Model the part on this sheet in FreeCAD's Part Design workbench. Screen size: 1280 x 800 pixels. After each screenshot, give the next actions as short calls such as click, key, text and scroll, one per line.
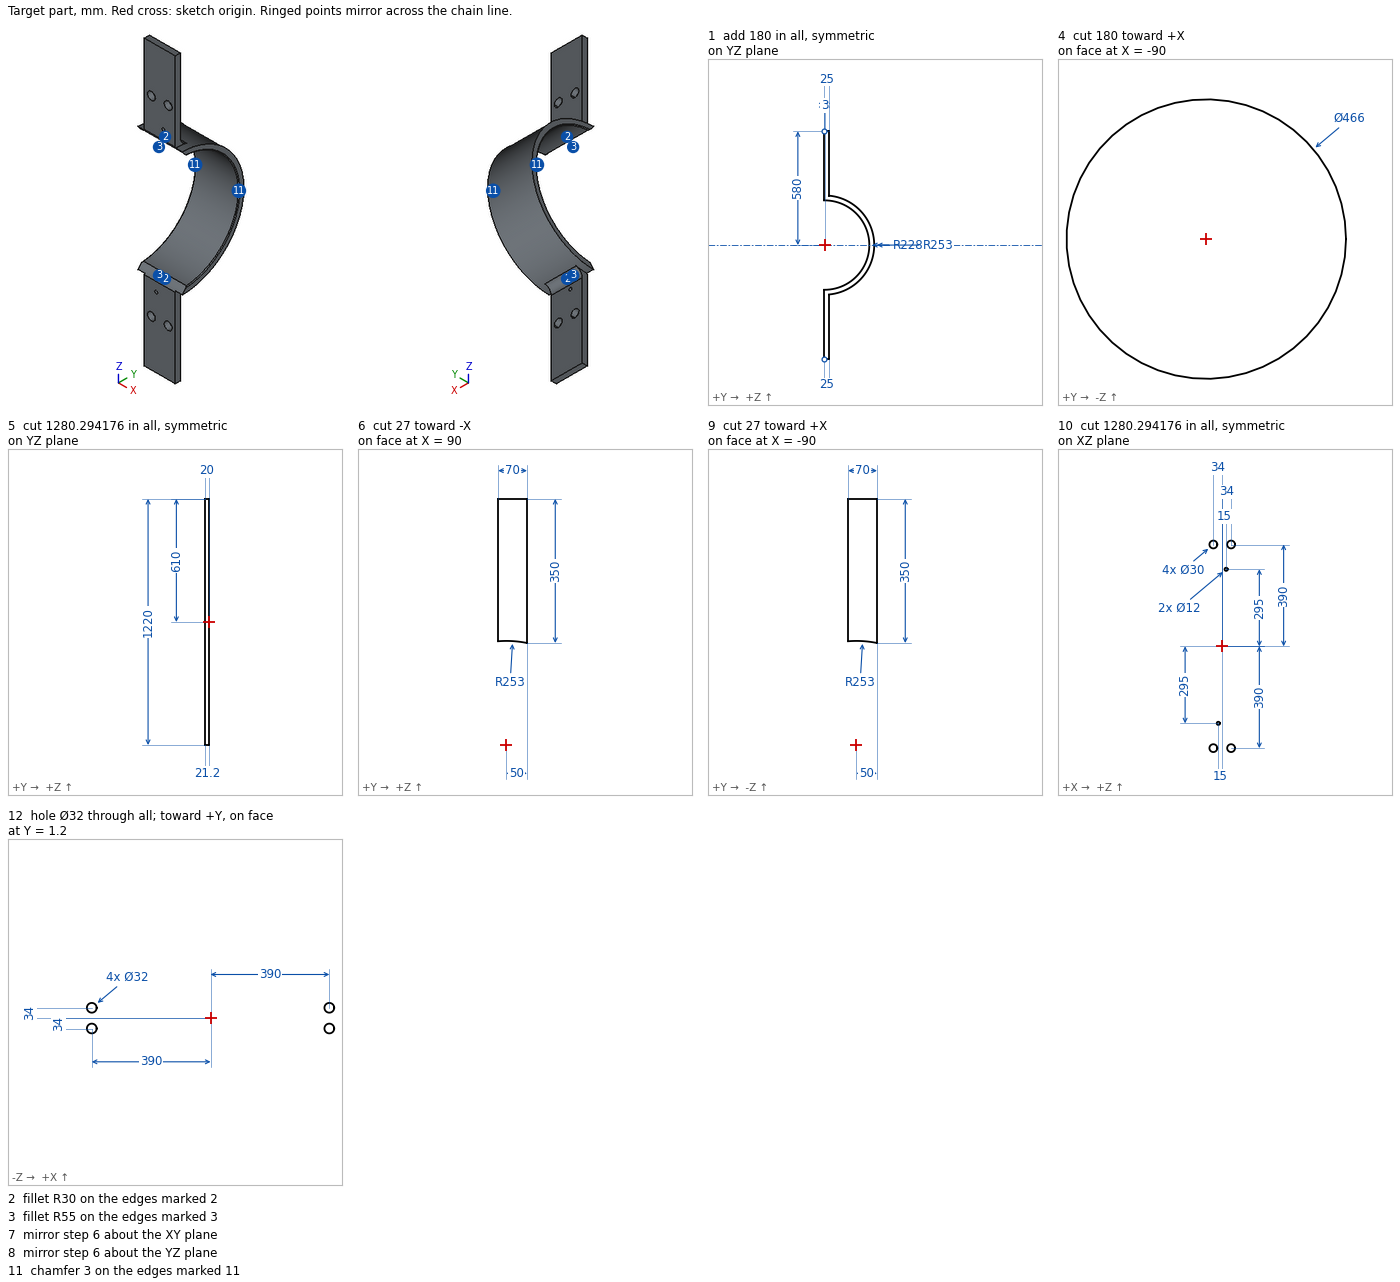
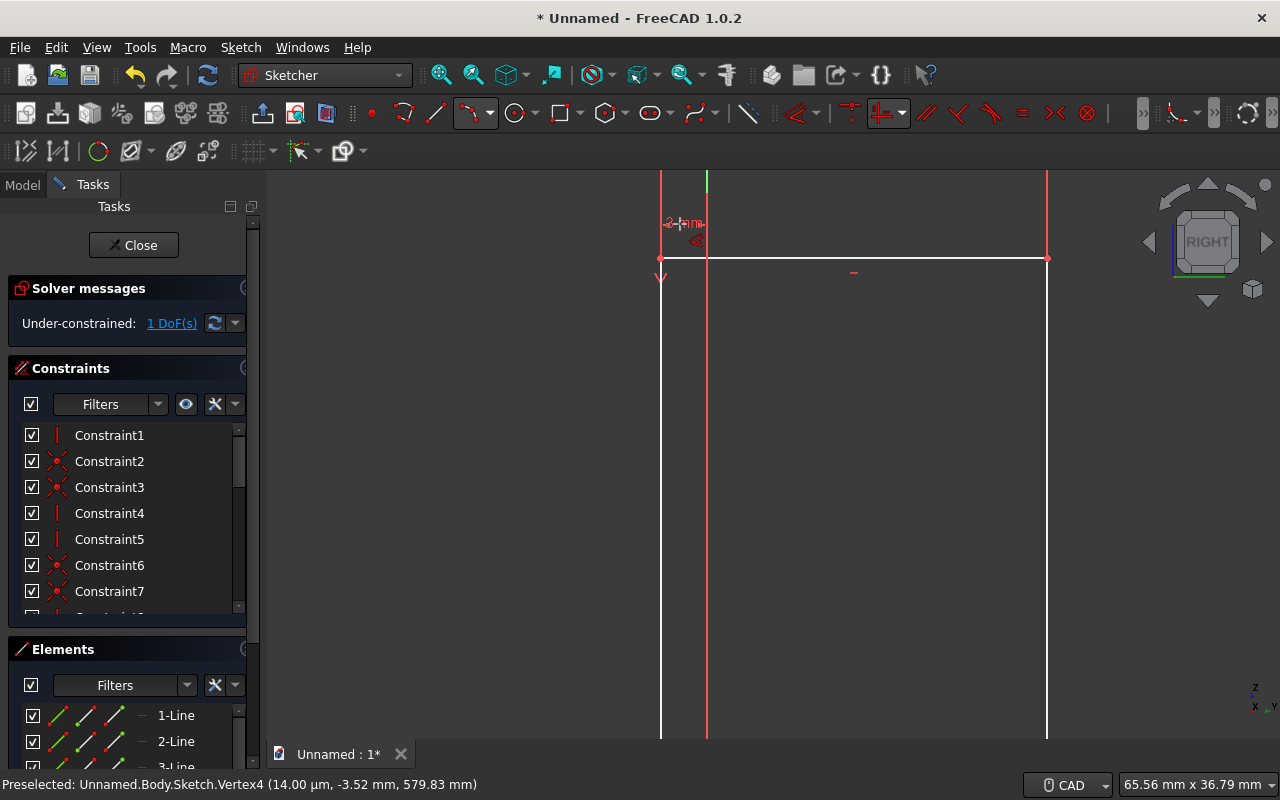
scroll(704, 454, down, 15)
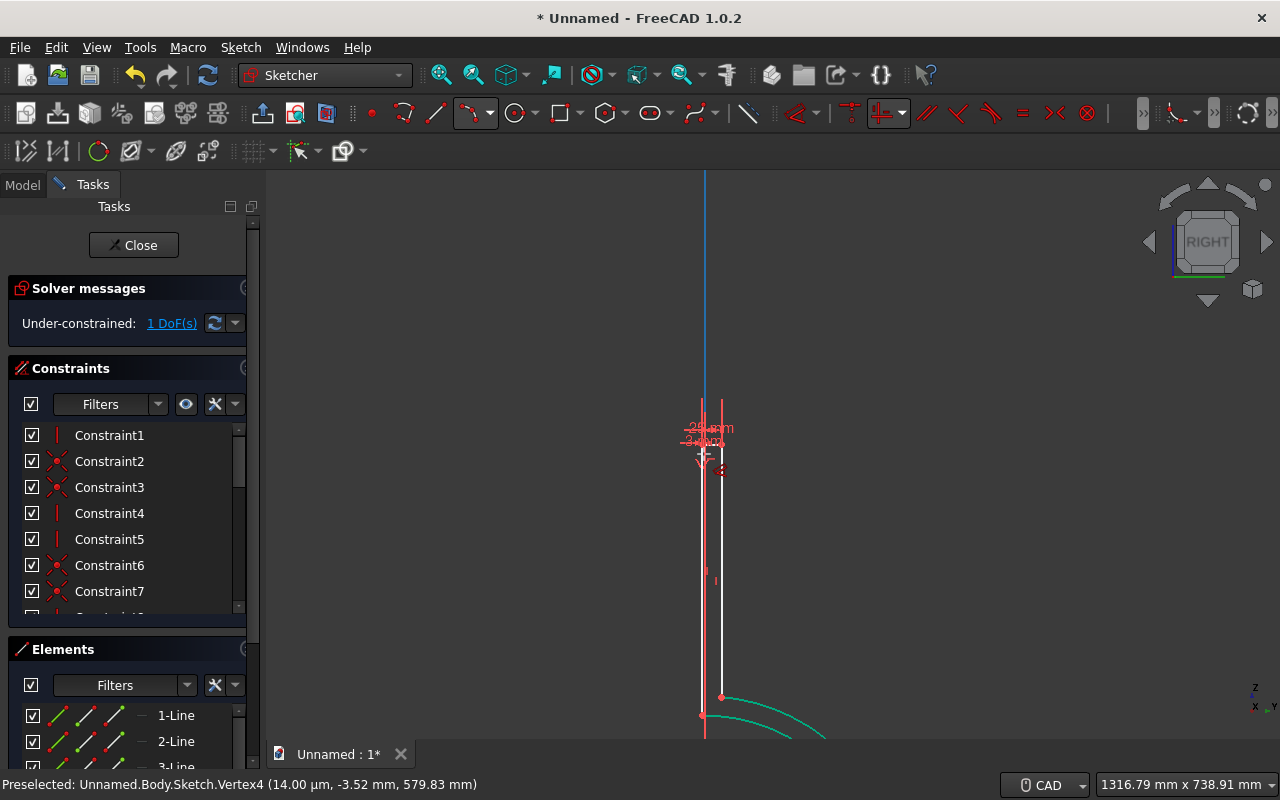
scroll(648, 200, down, 5)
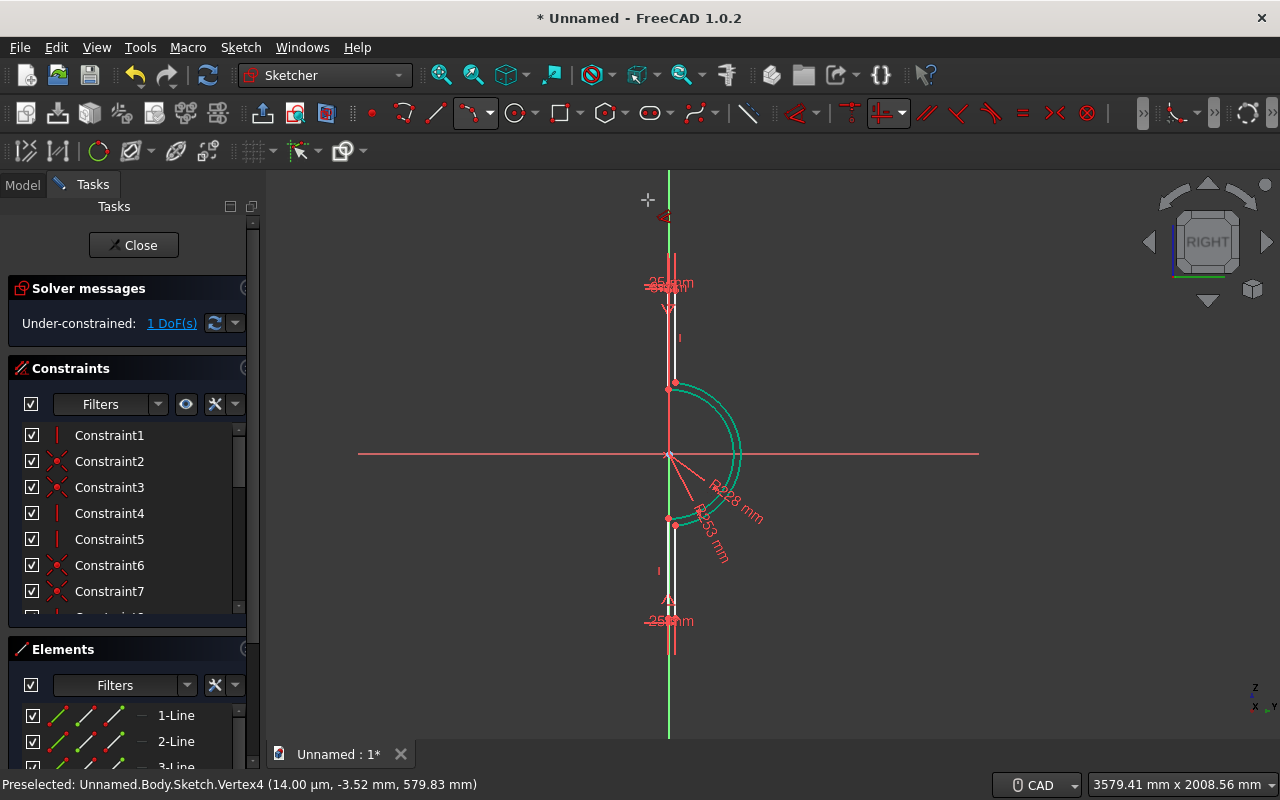
scroll(675, 290, up, 3)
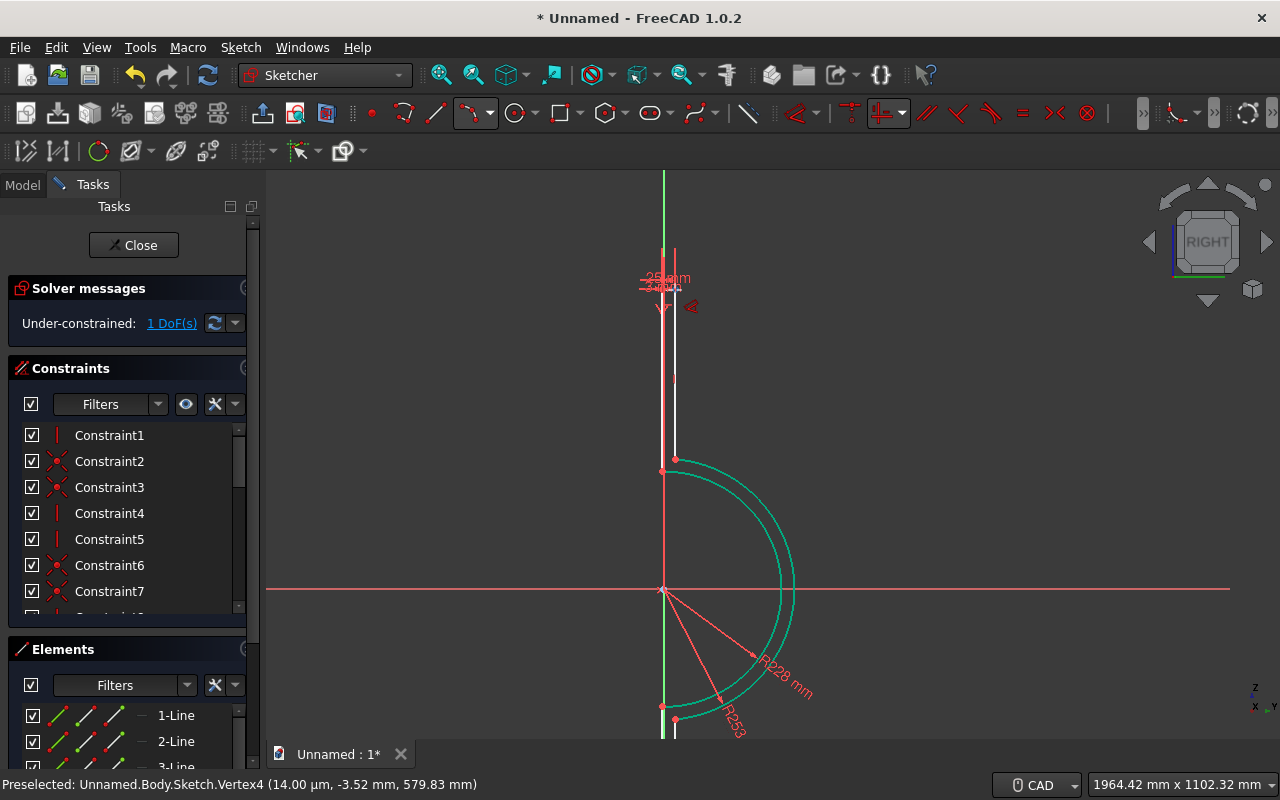
click(675, 290)
click(630, 440)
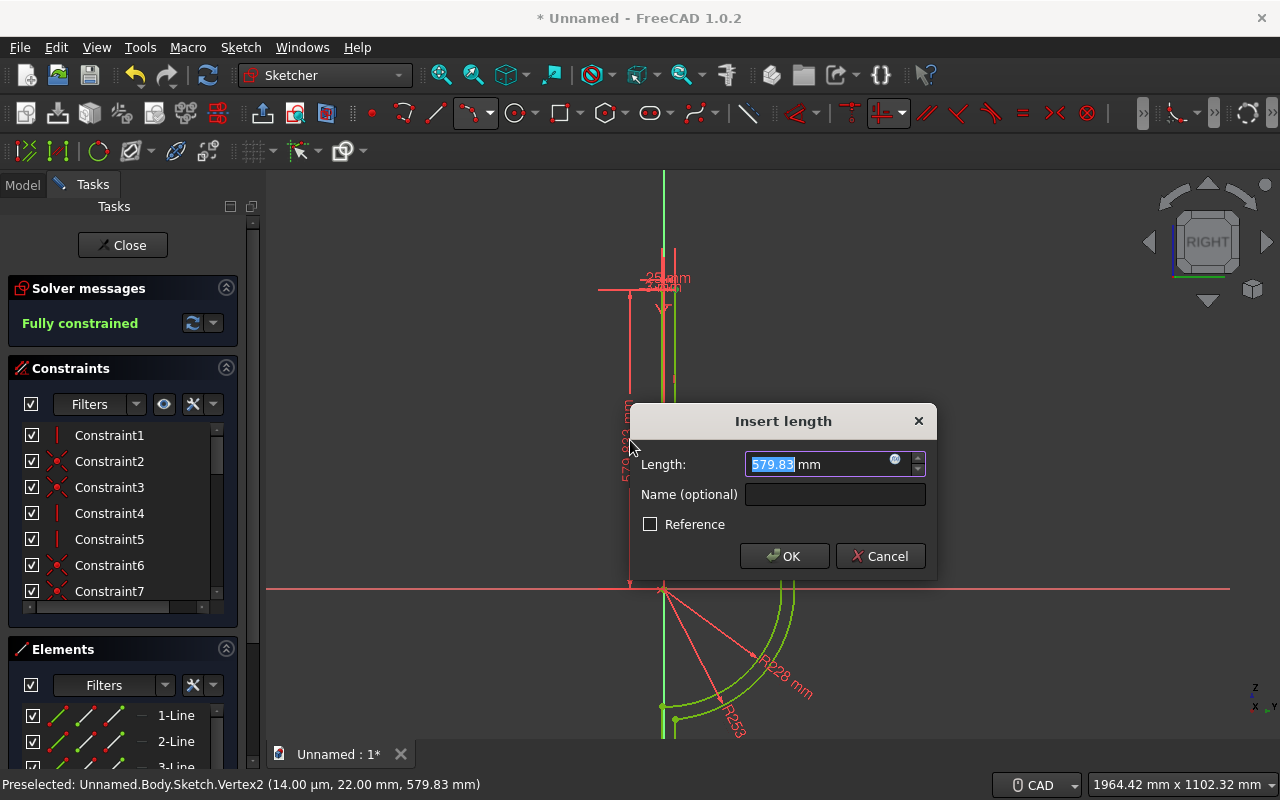
text(580)
key(Return)
key(Escape)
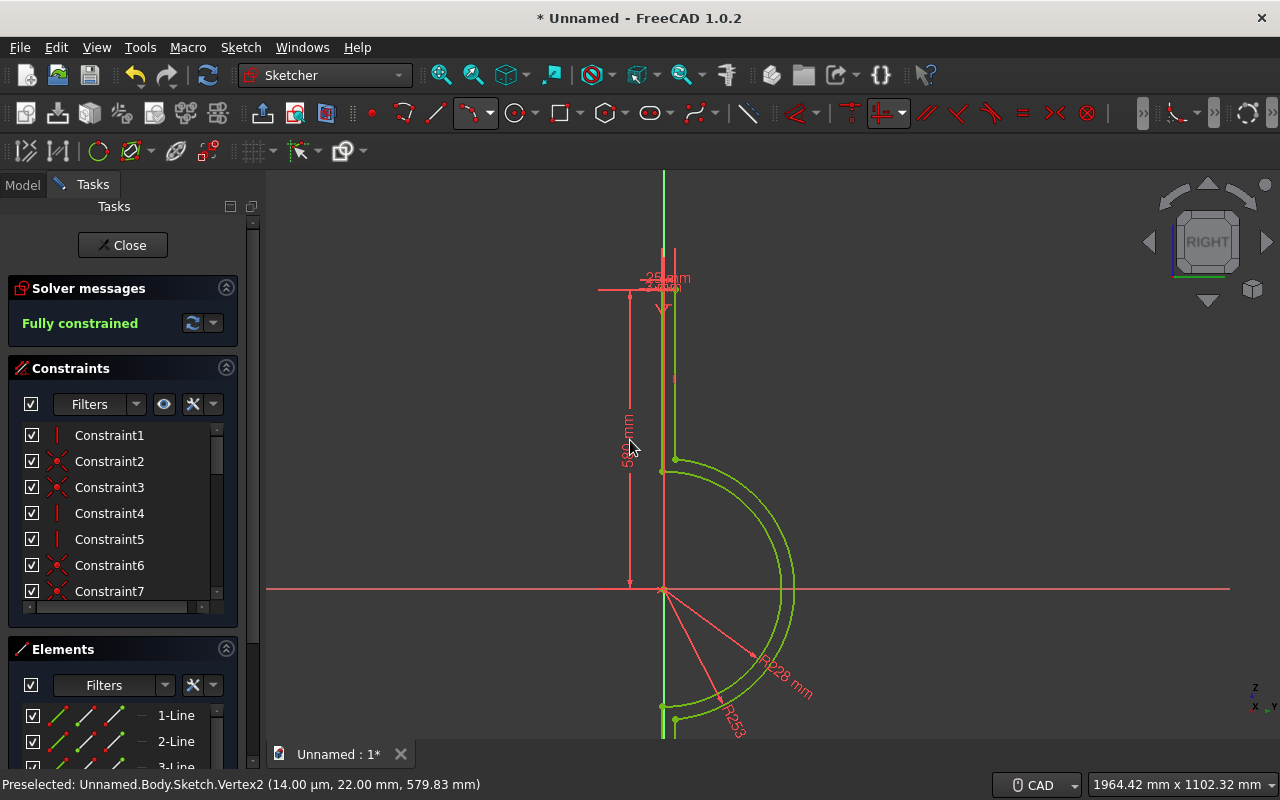
click(123, 245)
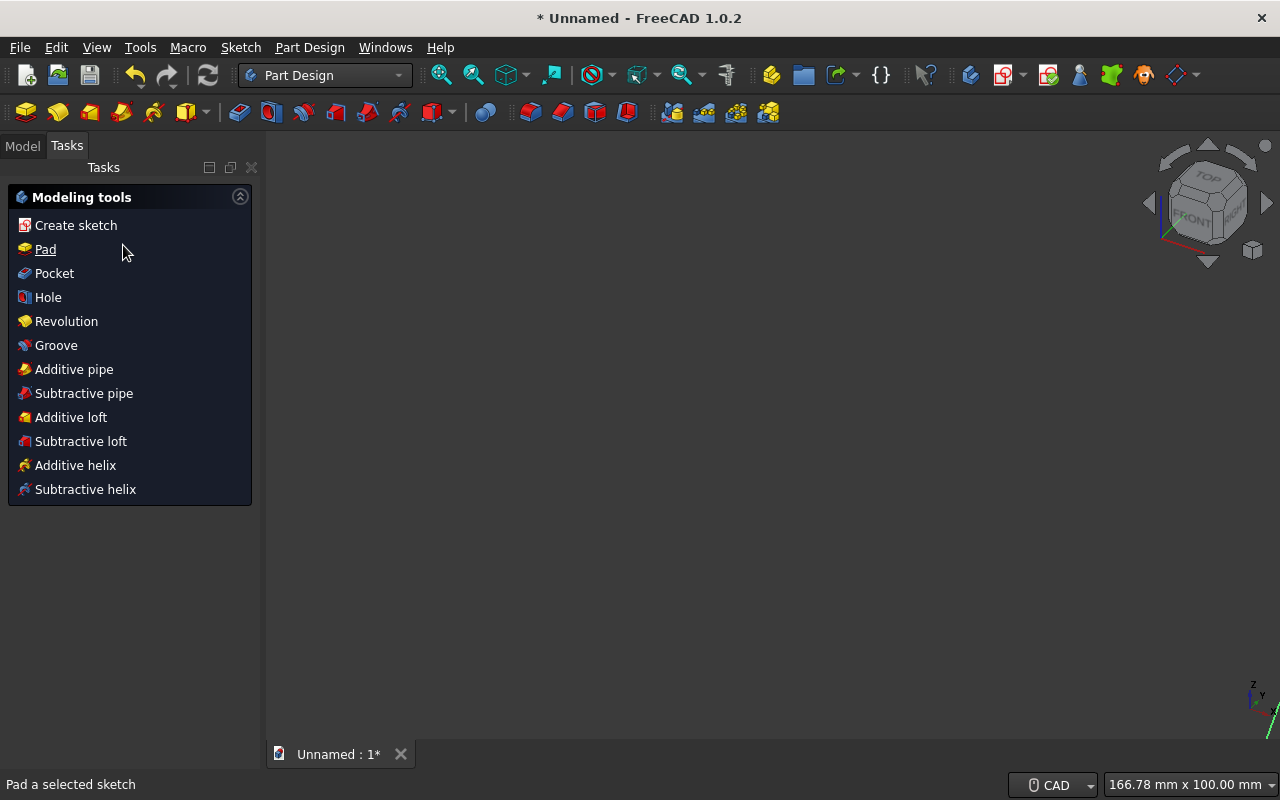
click(26, 112)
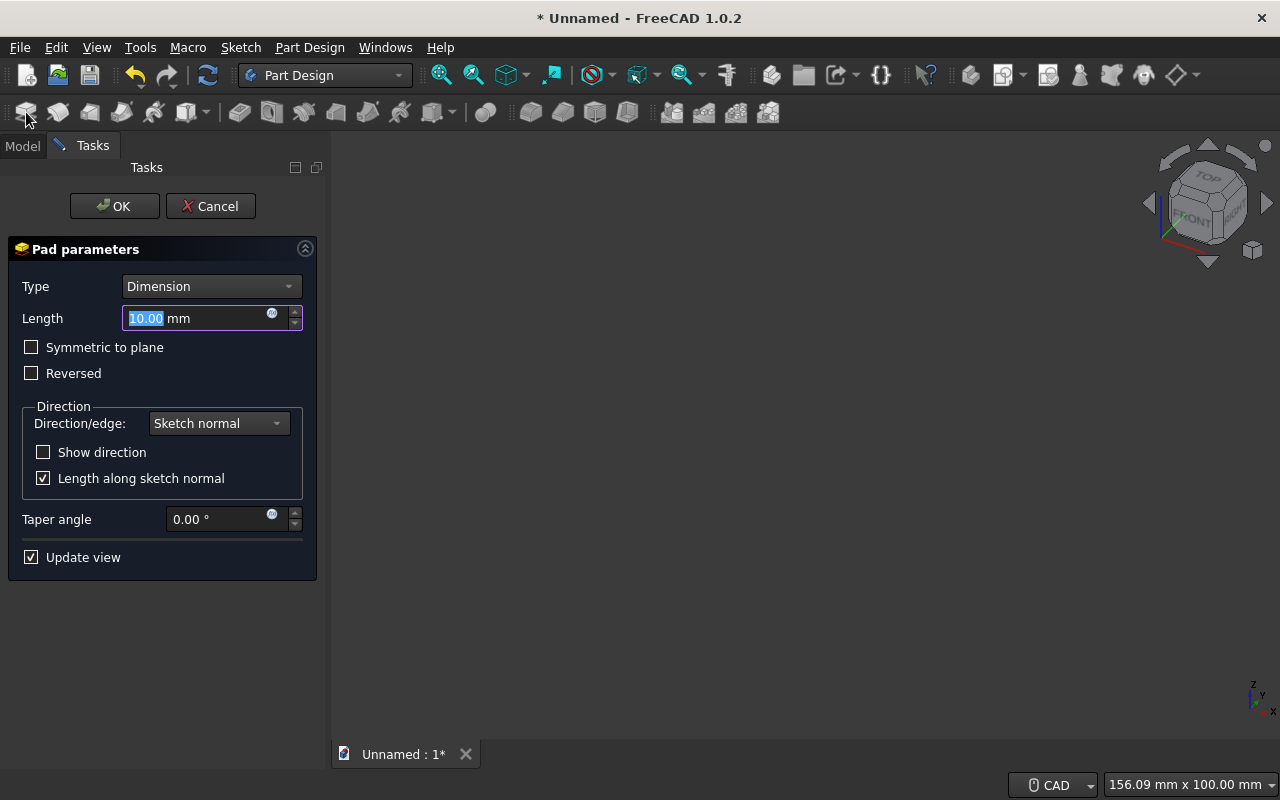
text(180)
key(Tab)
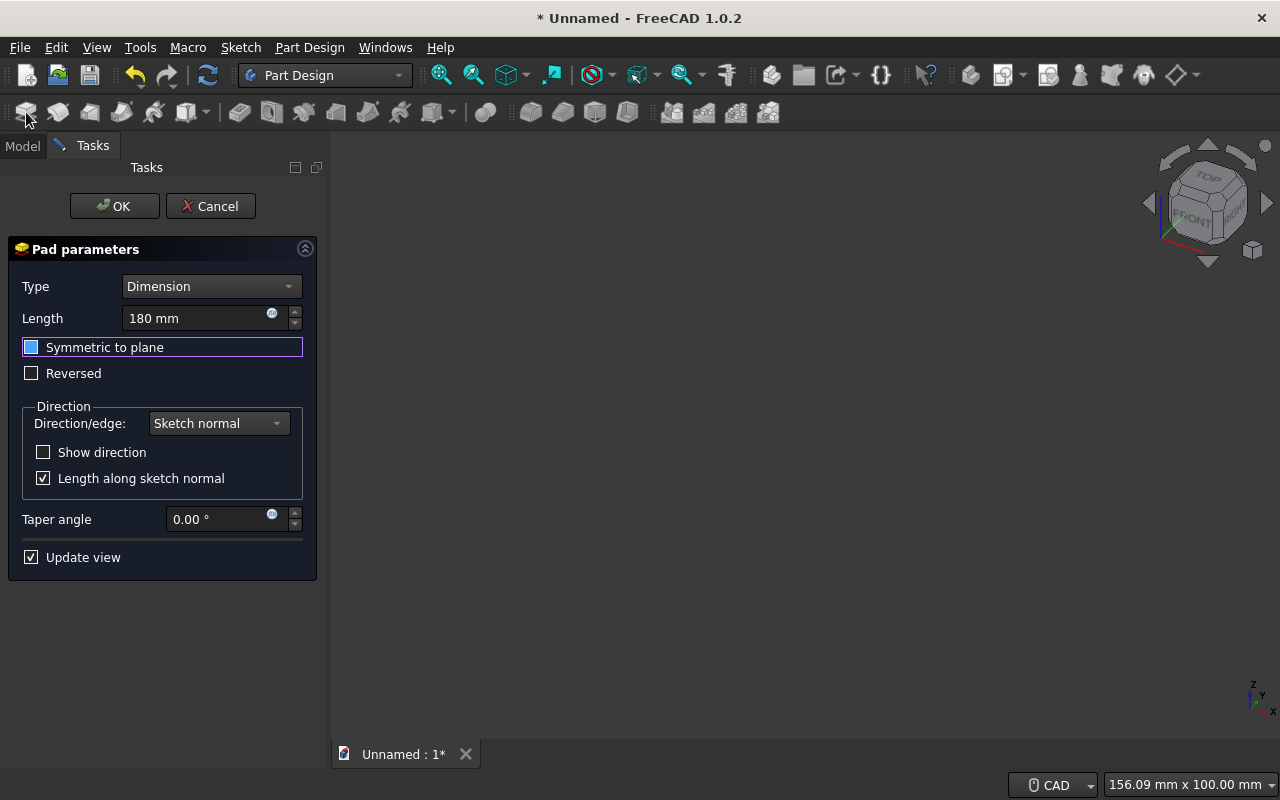
click(30, 347)